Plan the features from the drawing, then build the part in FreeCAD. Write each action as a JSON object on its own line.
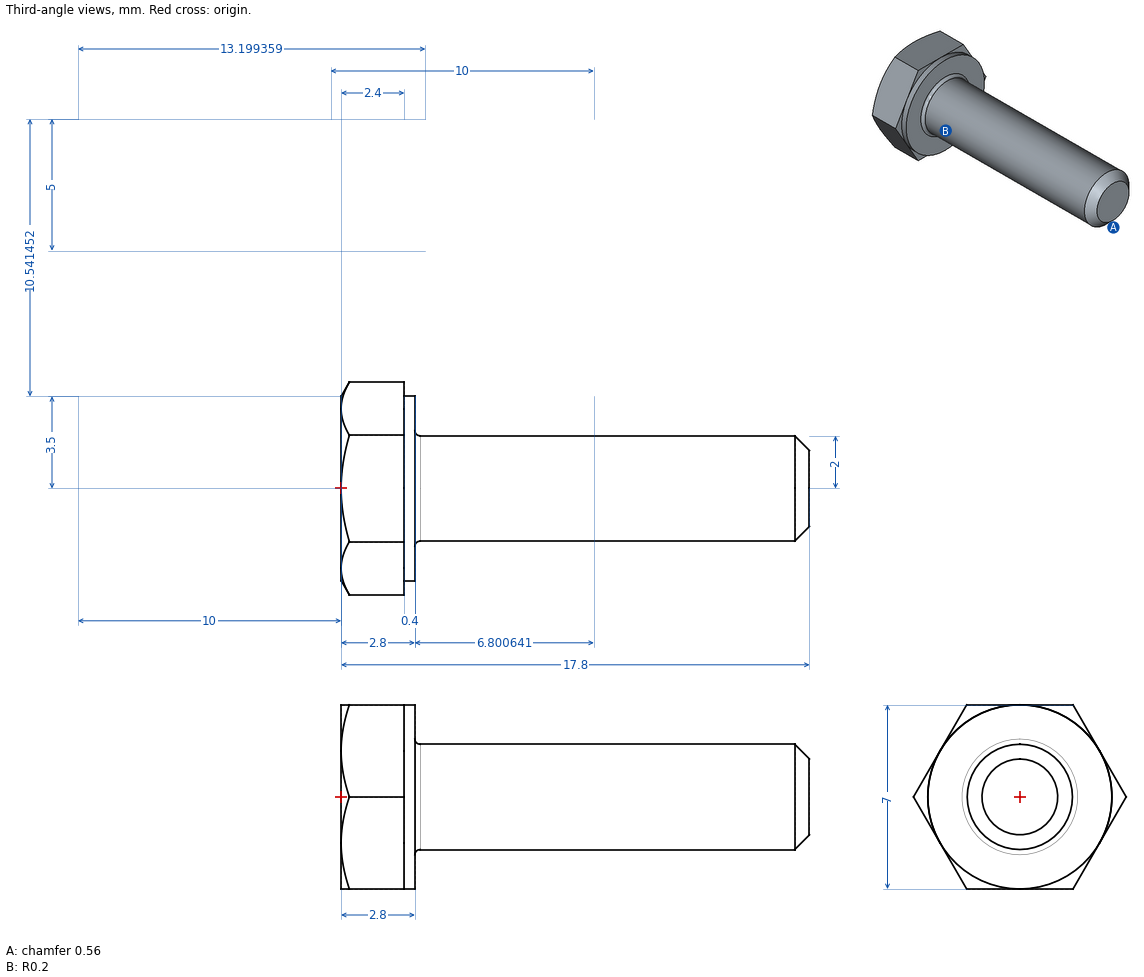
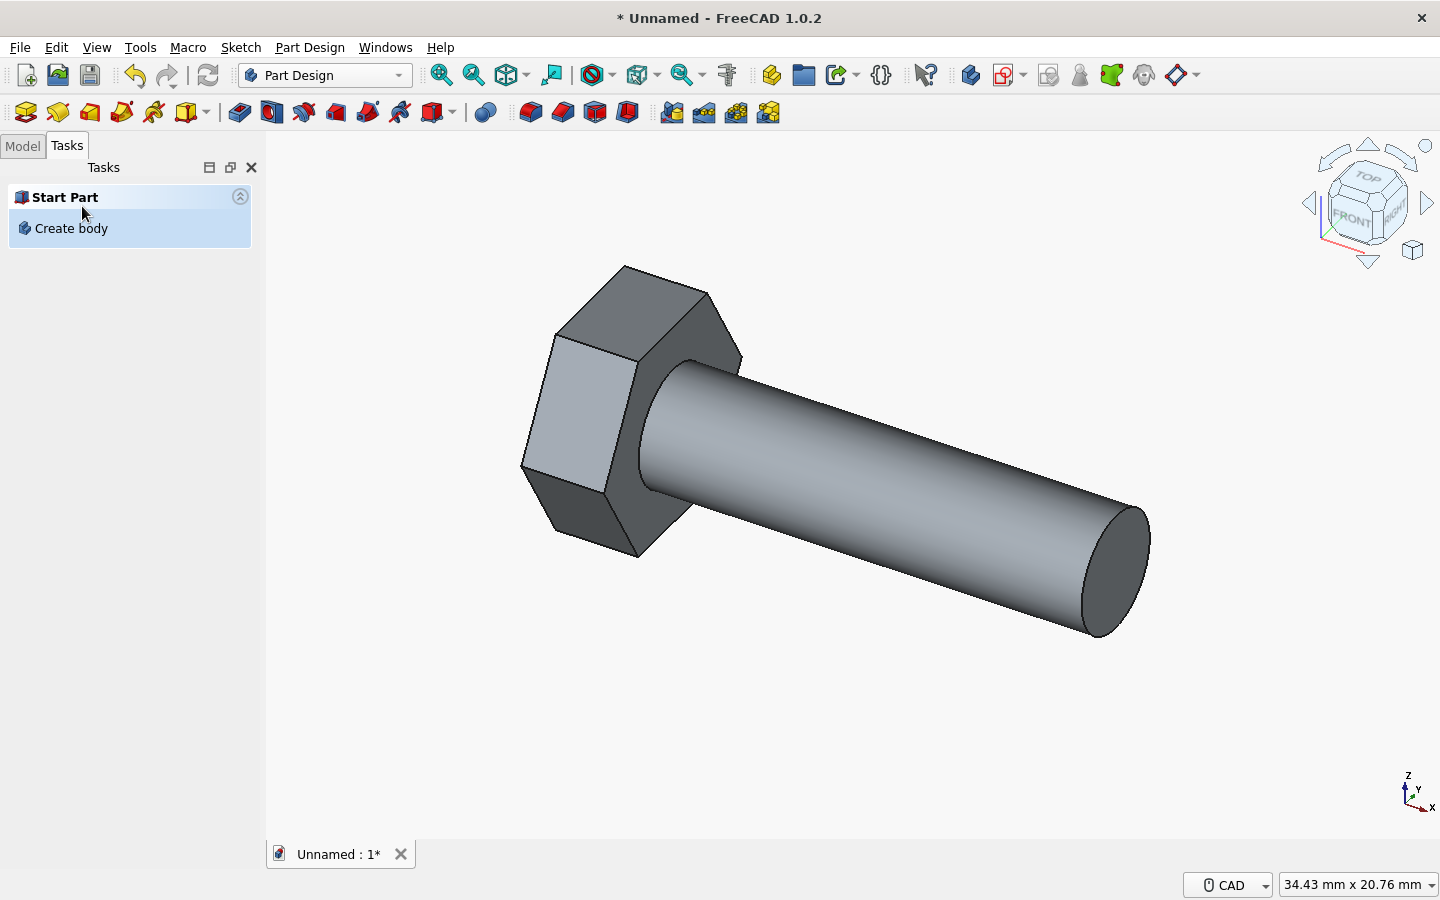
{"action": "left_click", "coordinate": [1004, 76]}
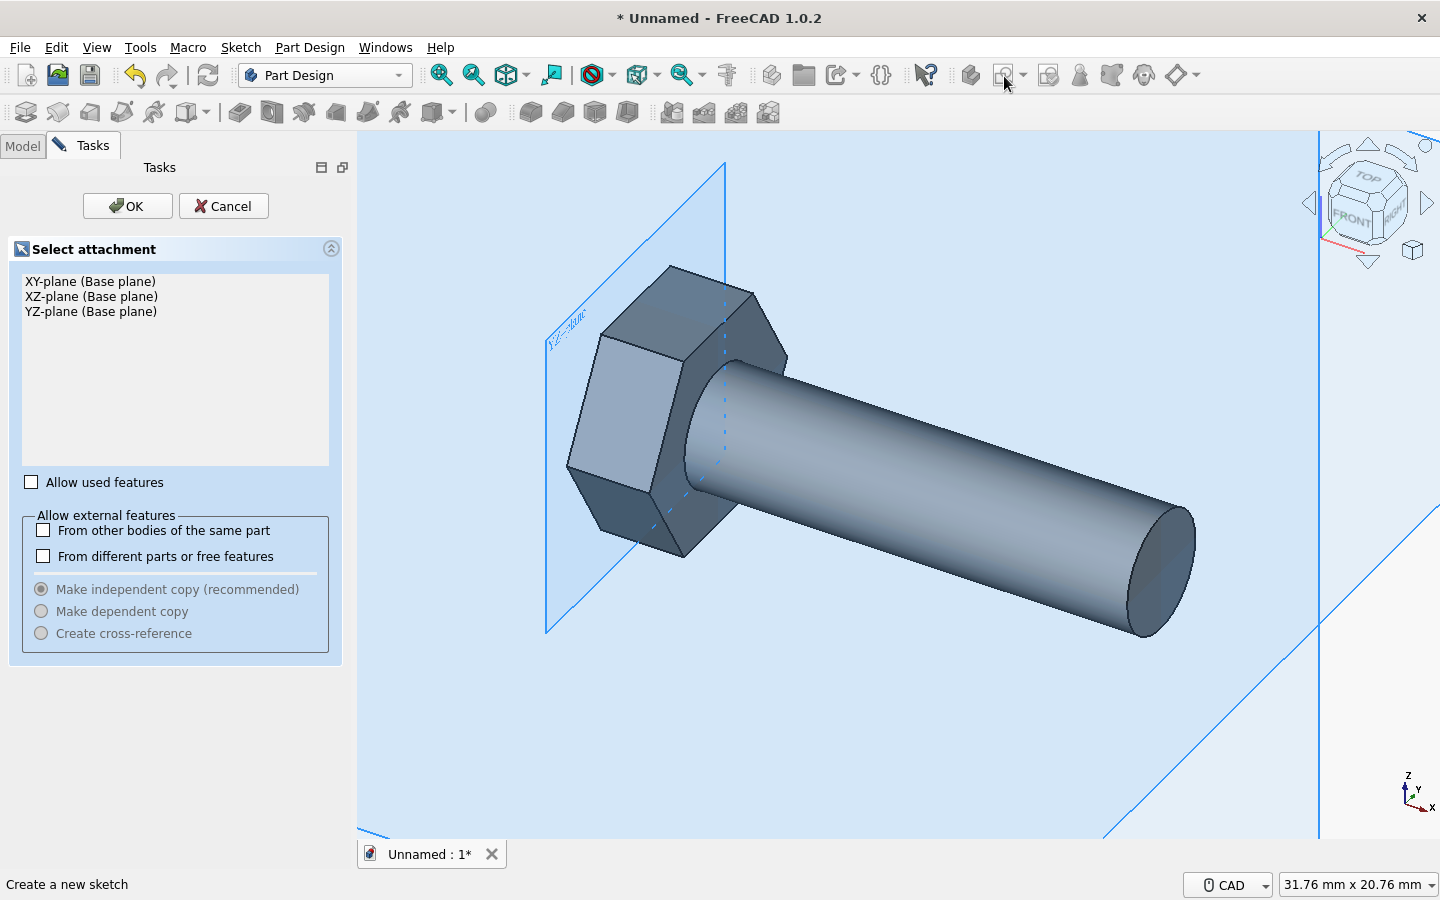
{"action": "left_click", "coordinate": [82, 282]}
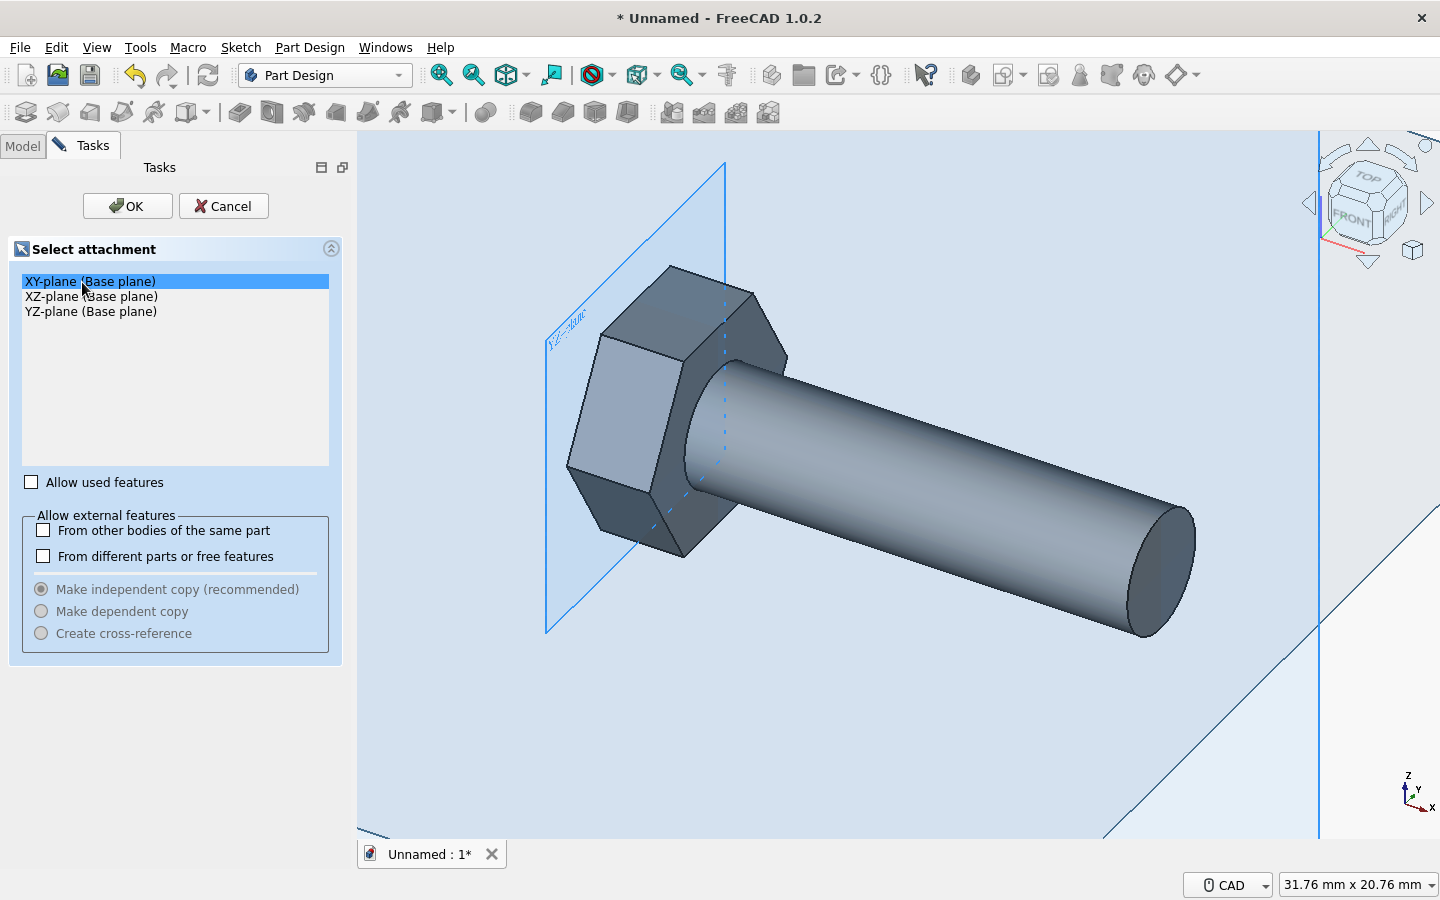
{"action": "left_click", "coordinate": [128, 206]}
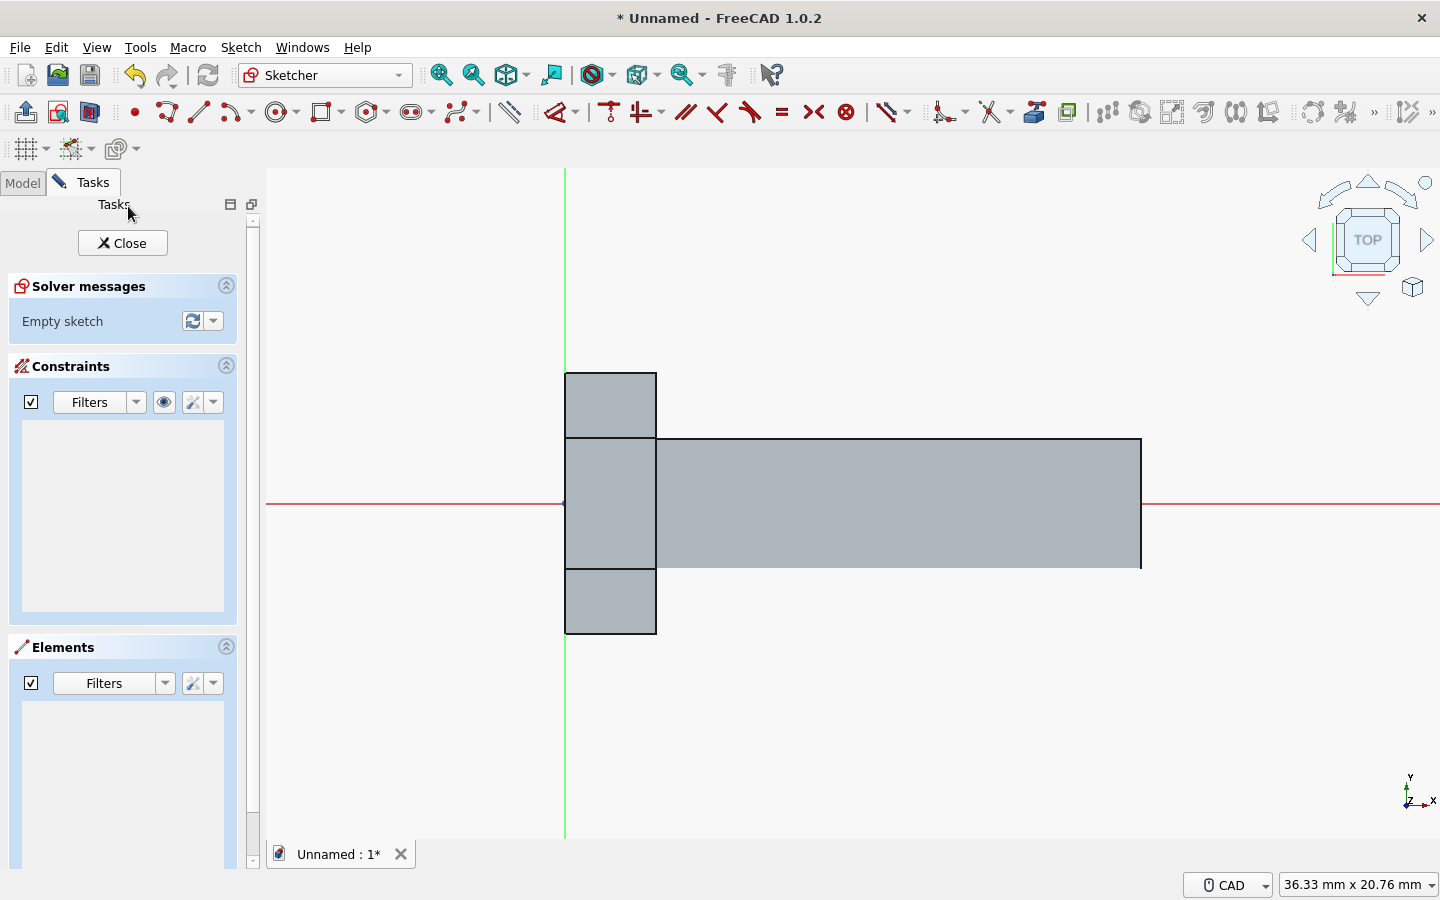
{"action": "key", "text": "q s"}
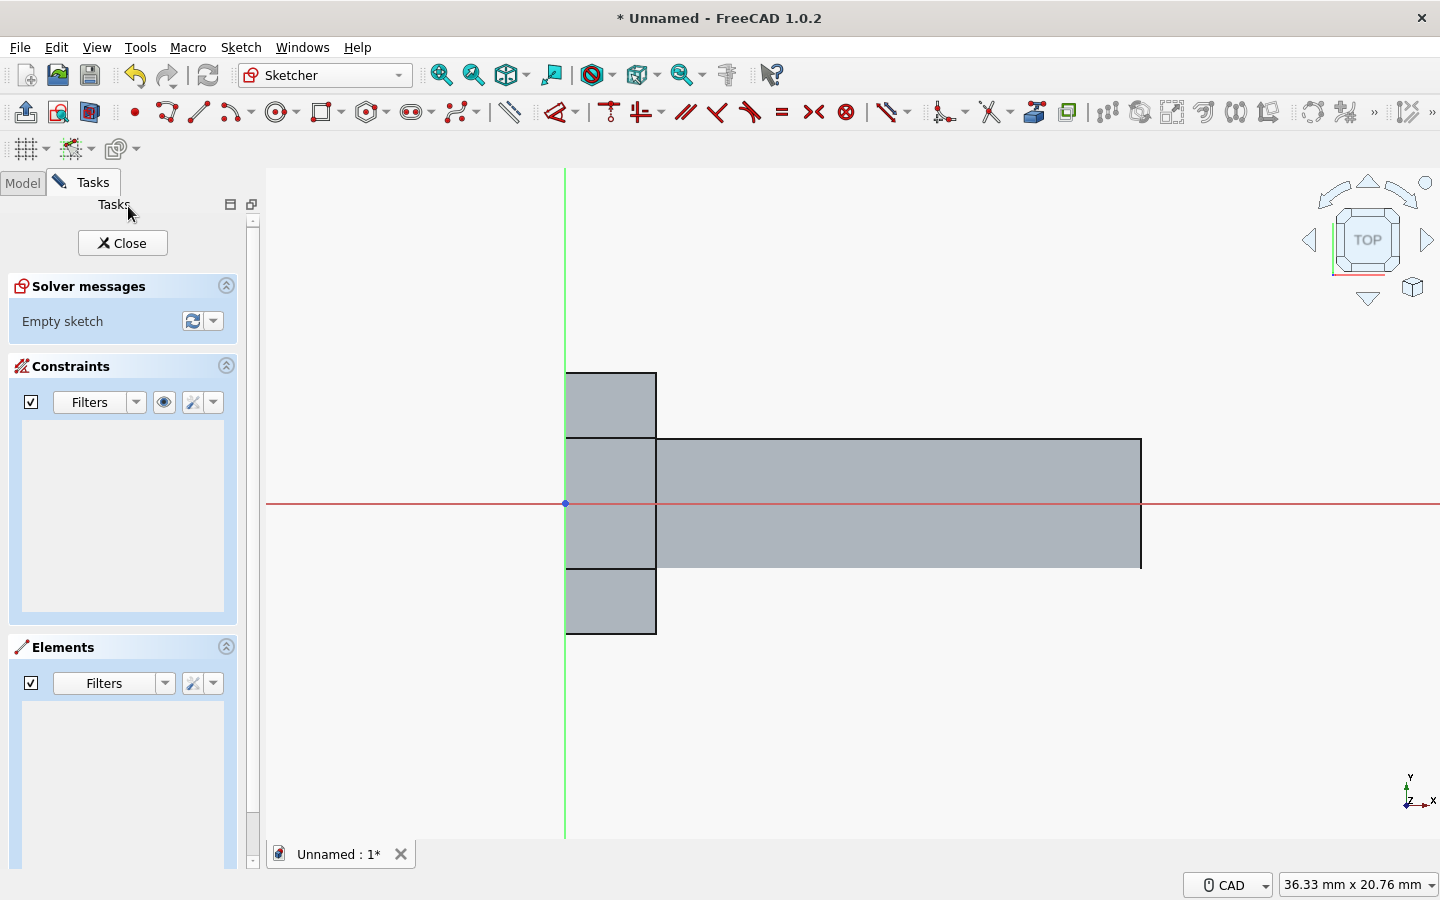
{"action": "scroll", "coordinate": [1275, 811], "scroll_direction": "down", "scroll_amount": 2}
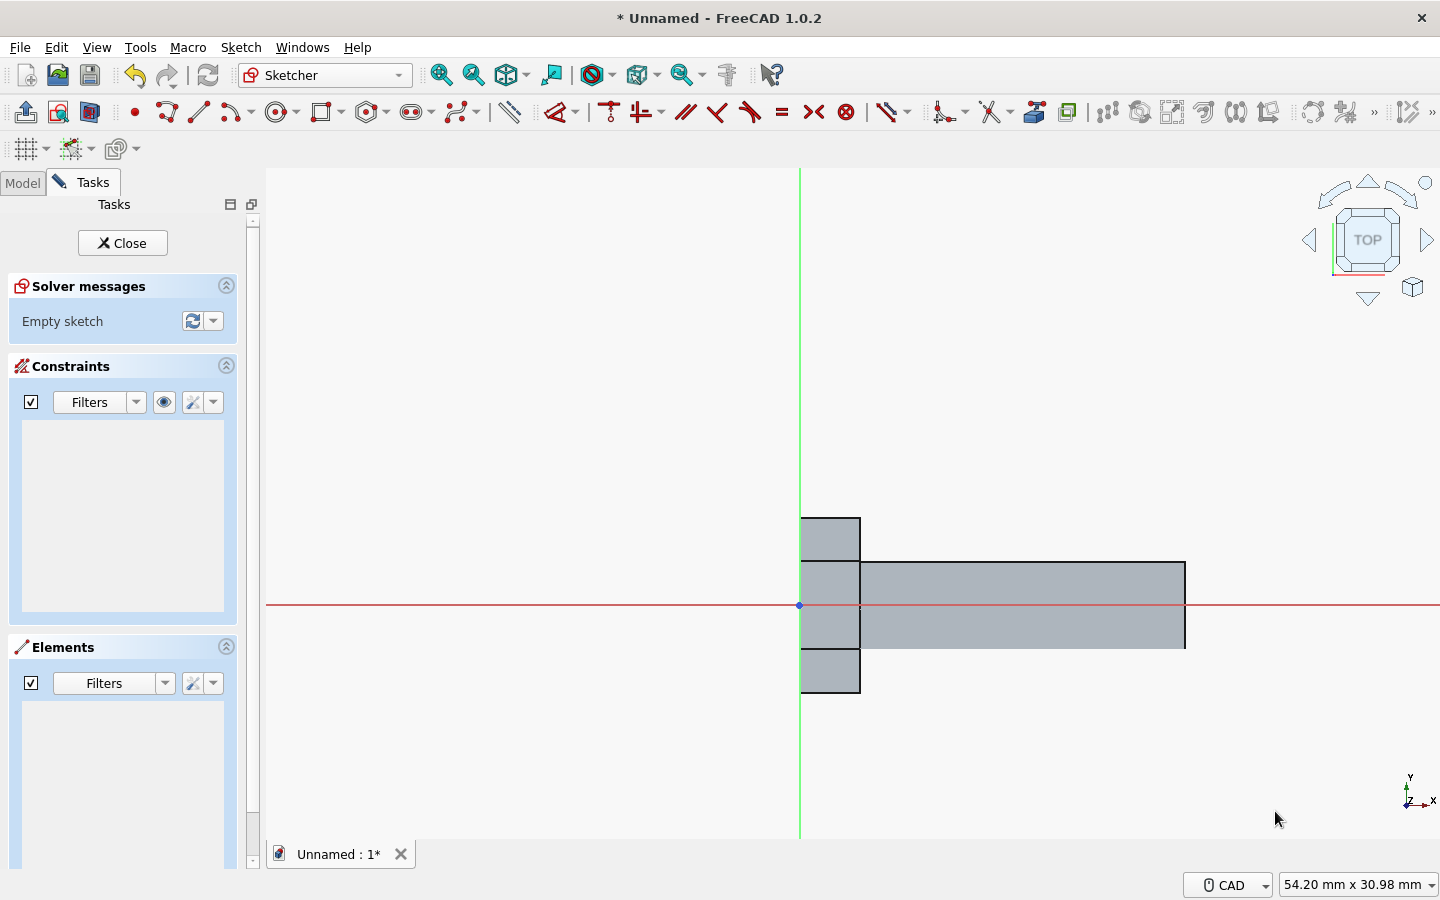
{"action": "scroll", "coordinate": [607, 351], "scroll_direction": "up", "scroll_amount": 2}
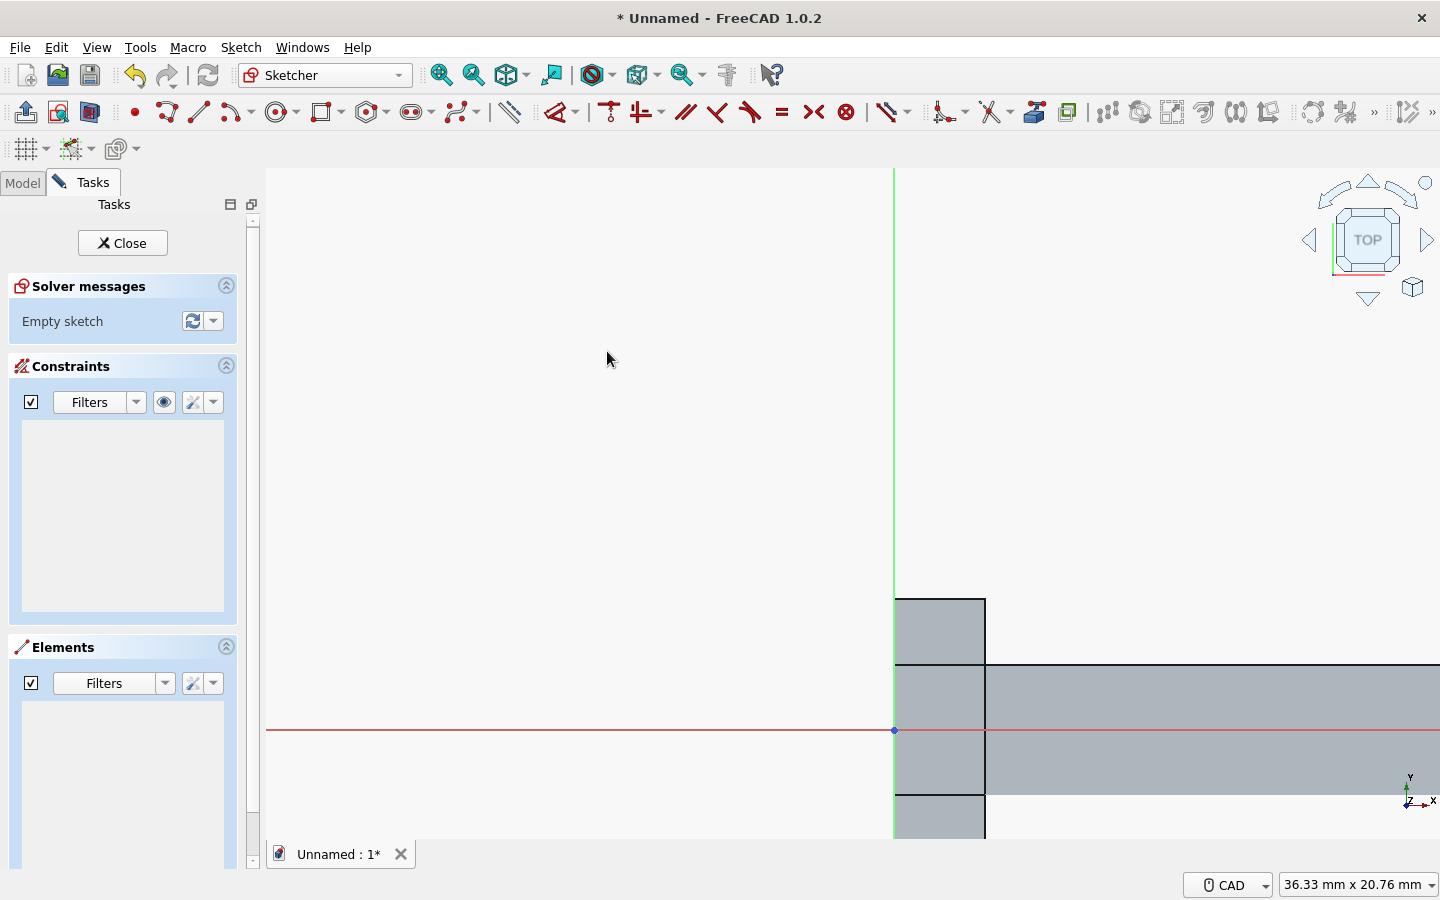
{"action": "left_click", "coordinate": [168, 112]}